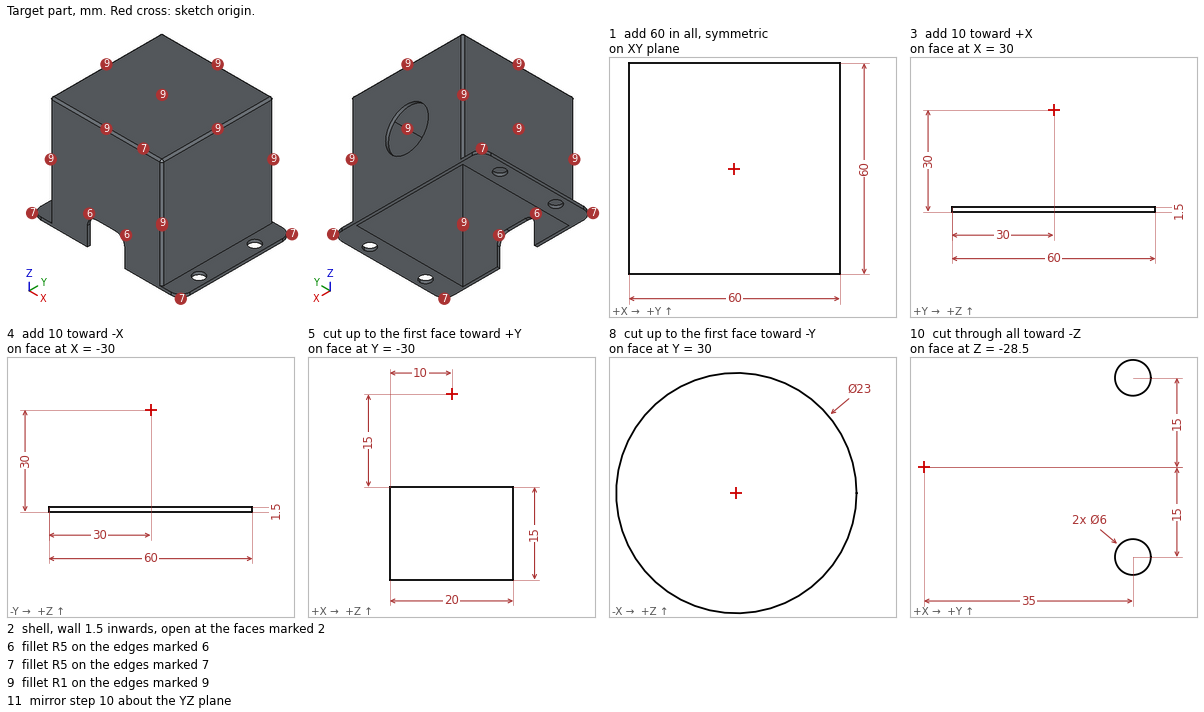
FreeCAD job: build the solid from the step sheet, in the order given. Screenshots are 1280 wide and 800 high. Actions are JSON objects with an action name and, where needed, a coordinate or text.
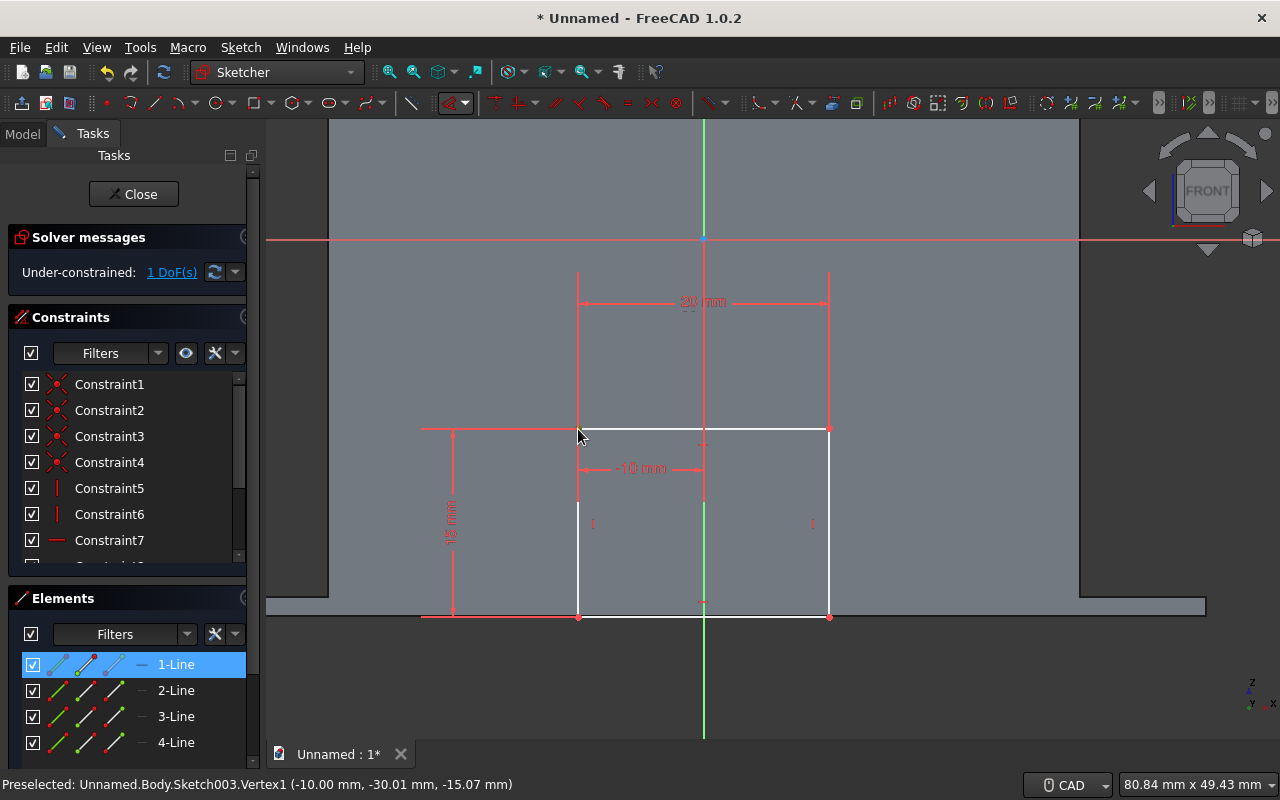
{"action": "left_click", "coordinate": [468, 104]}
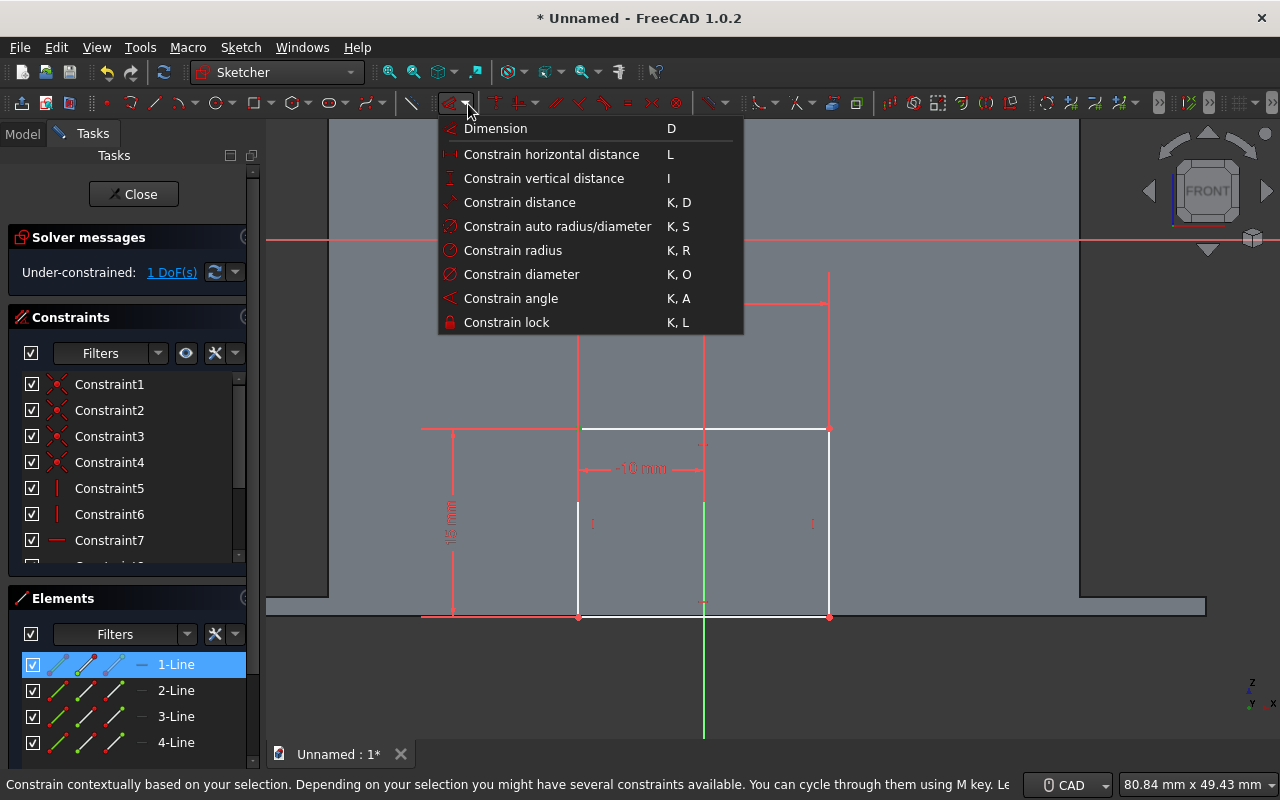
{"action": "left_click", "coordinate": [591, 178]}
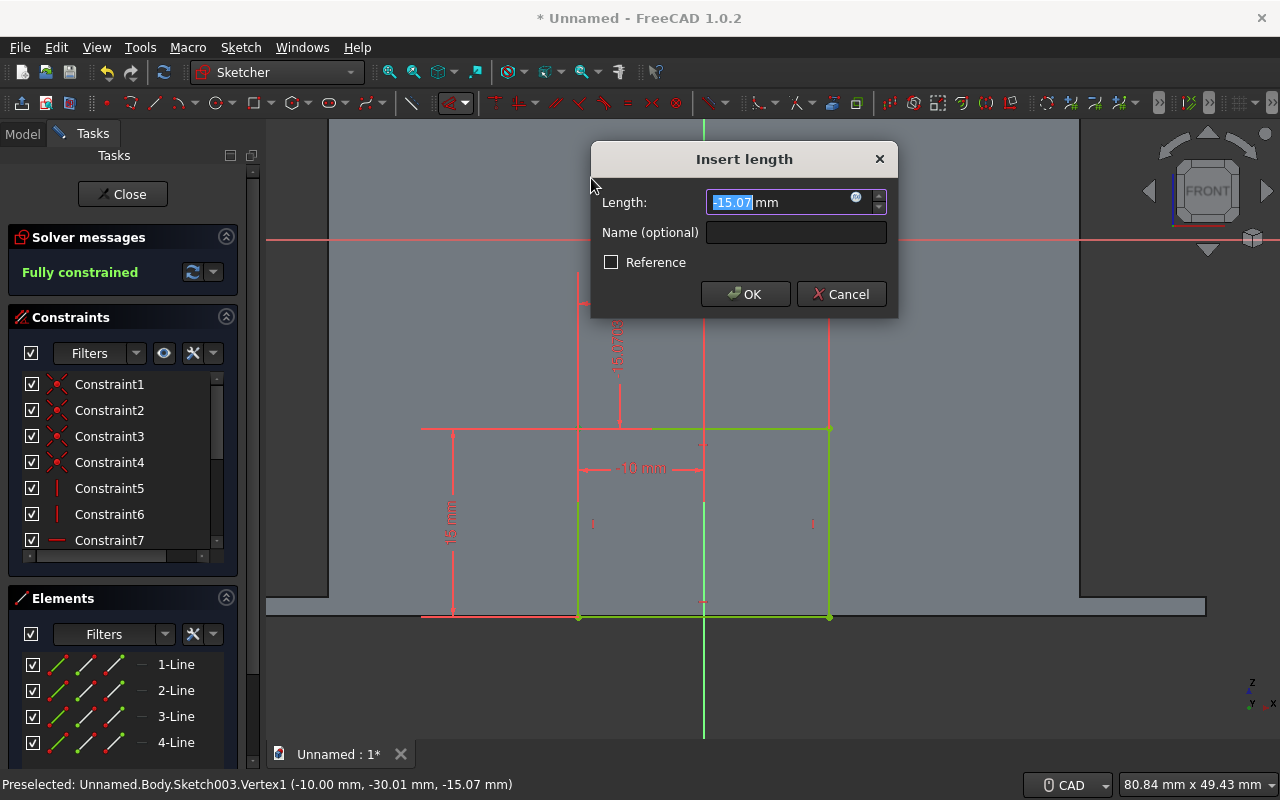
{"action": "type", "text": "-15"}
{"action": "key", "text": "Return"}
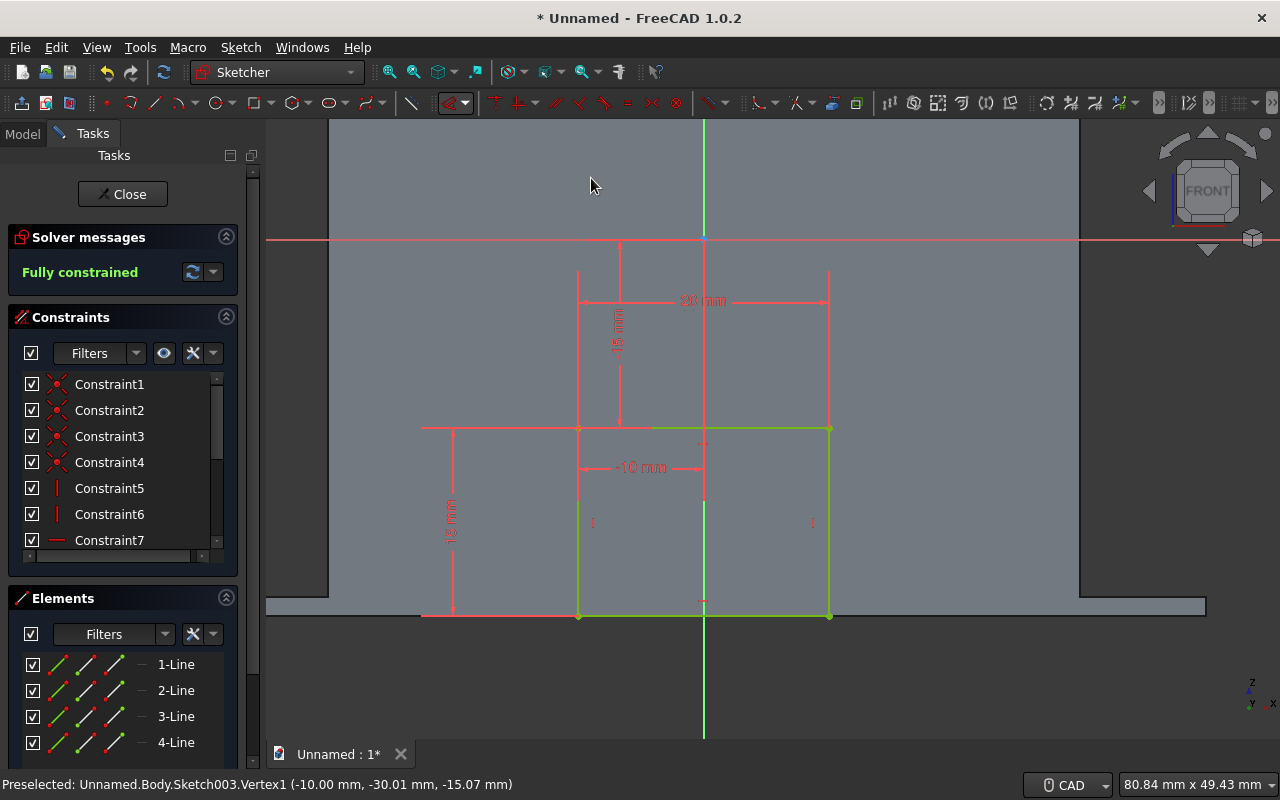
{"action": "left_click", "coordinate": [123, 194]}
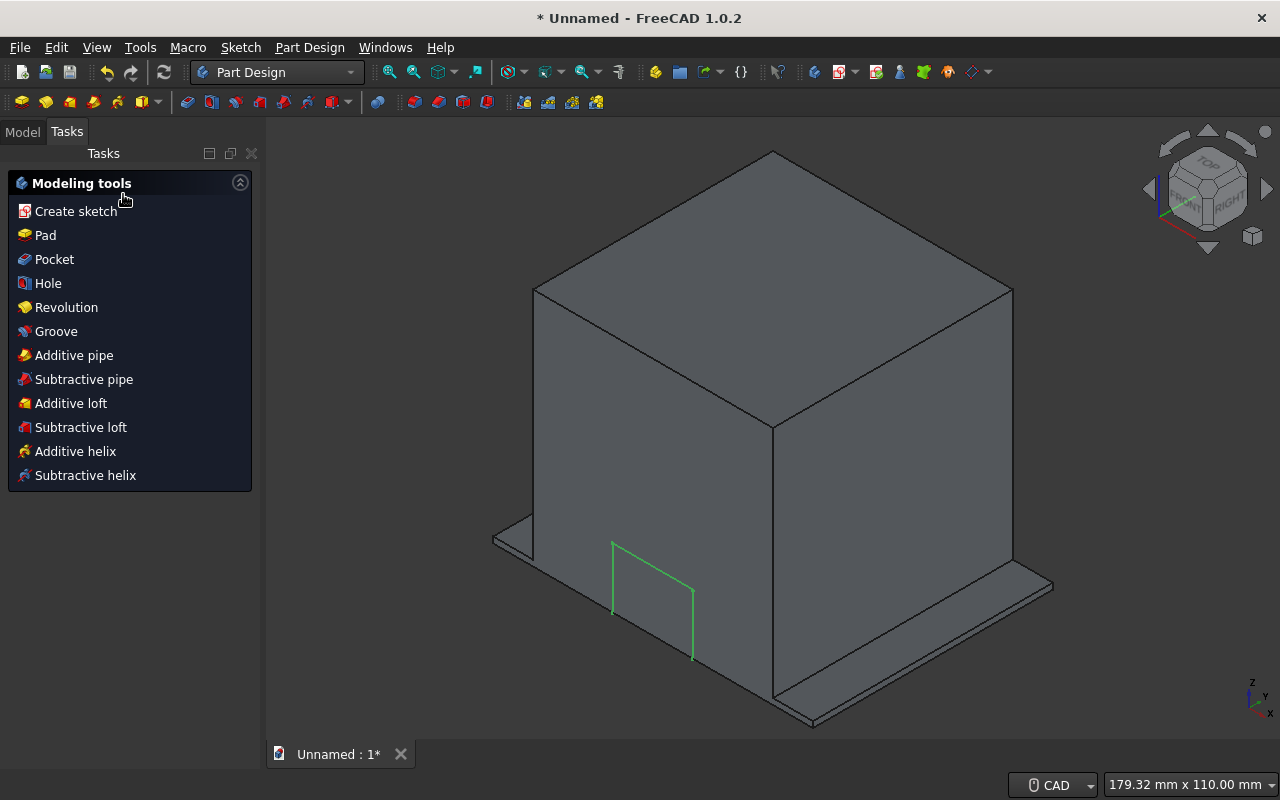
{"action": "left_click", "coordinate": [188, 102]}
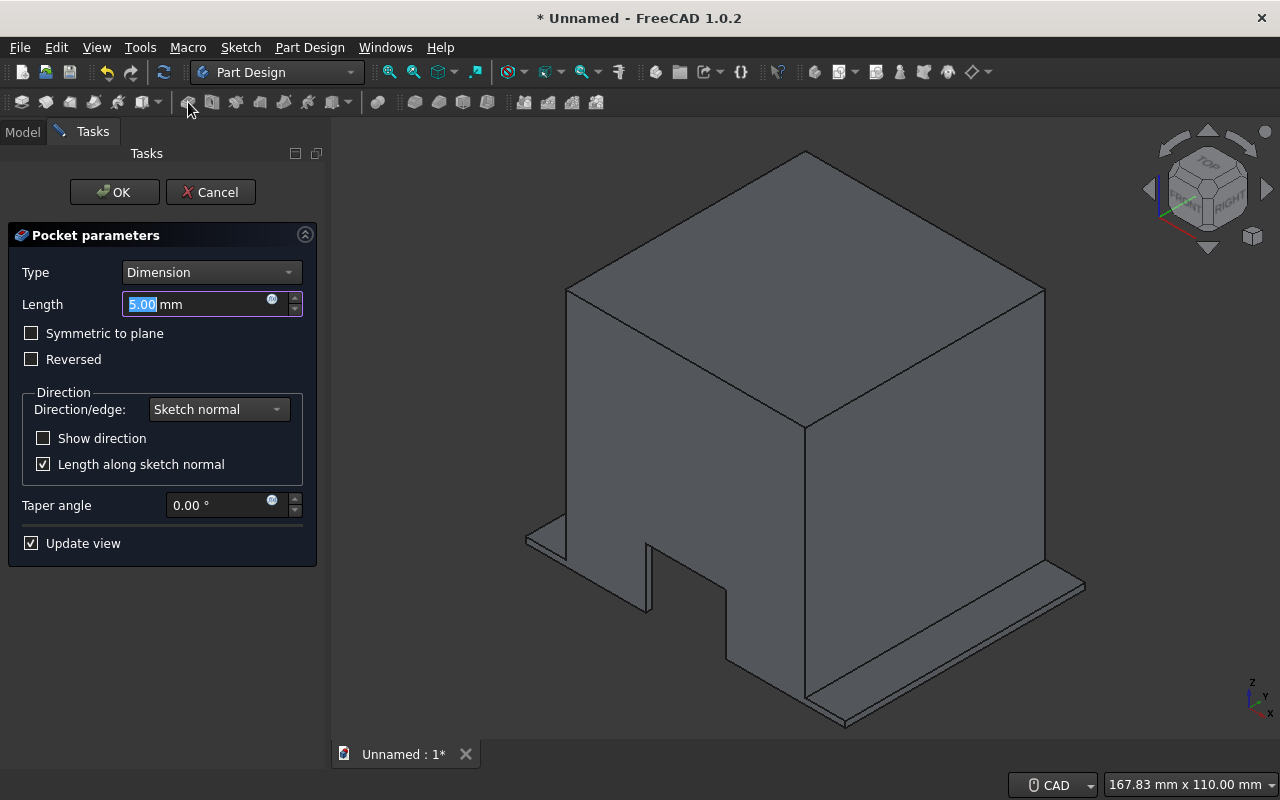
{"action": "left_click", "coordinate": [212, 272]}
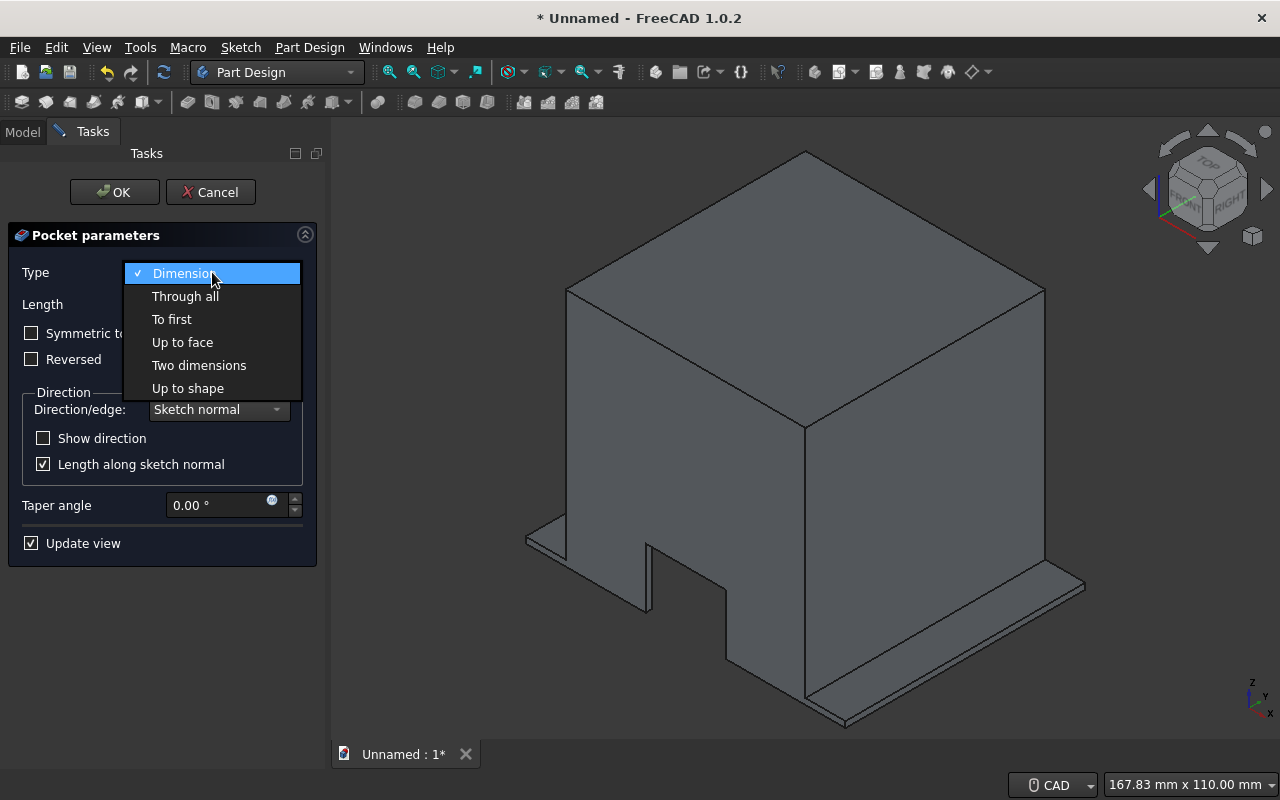
{"action": "left_click", "coordinate": [212, 320]}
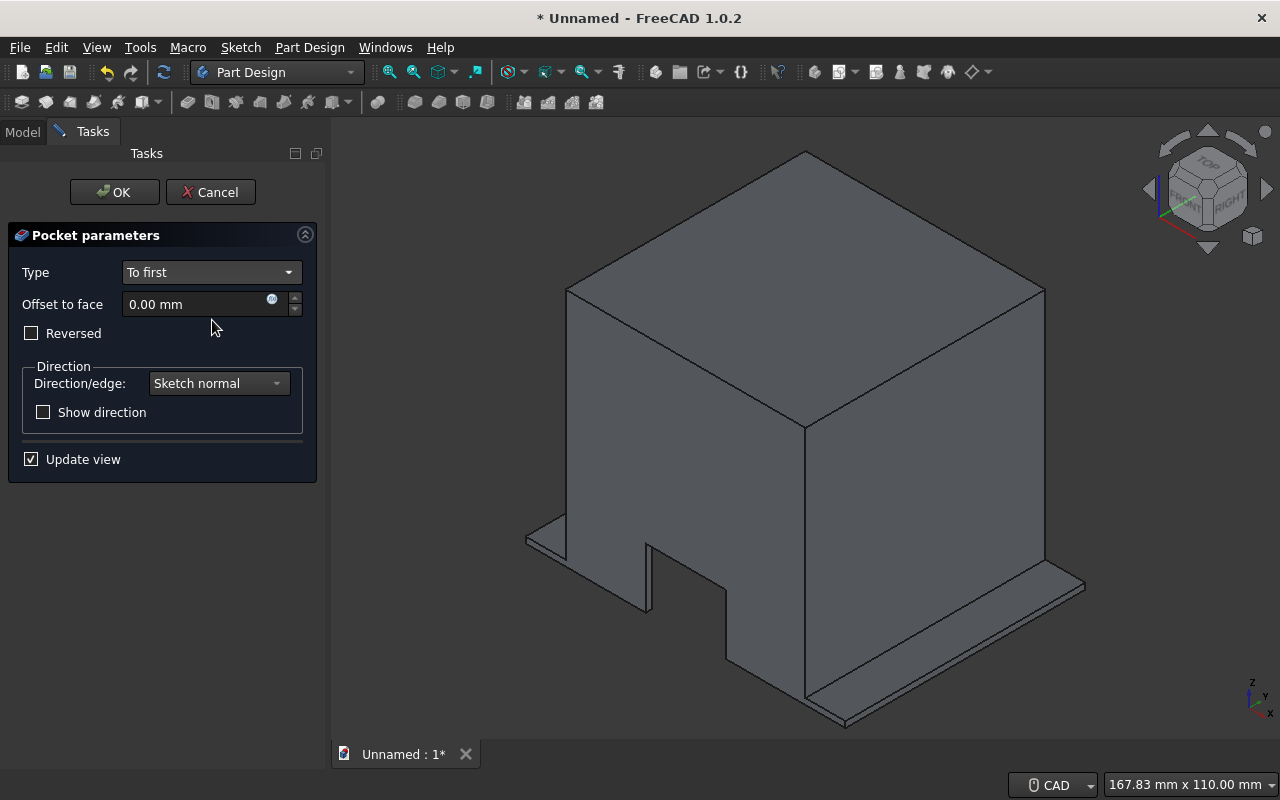
{"action": "left_click", "coordinate": [115, 192]}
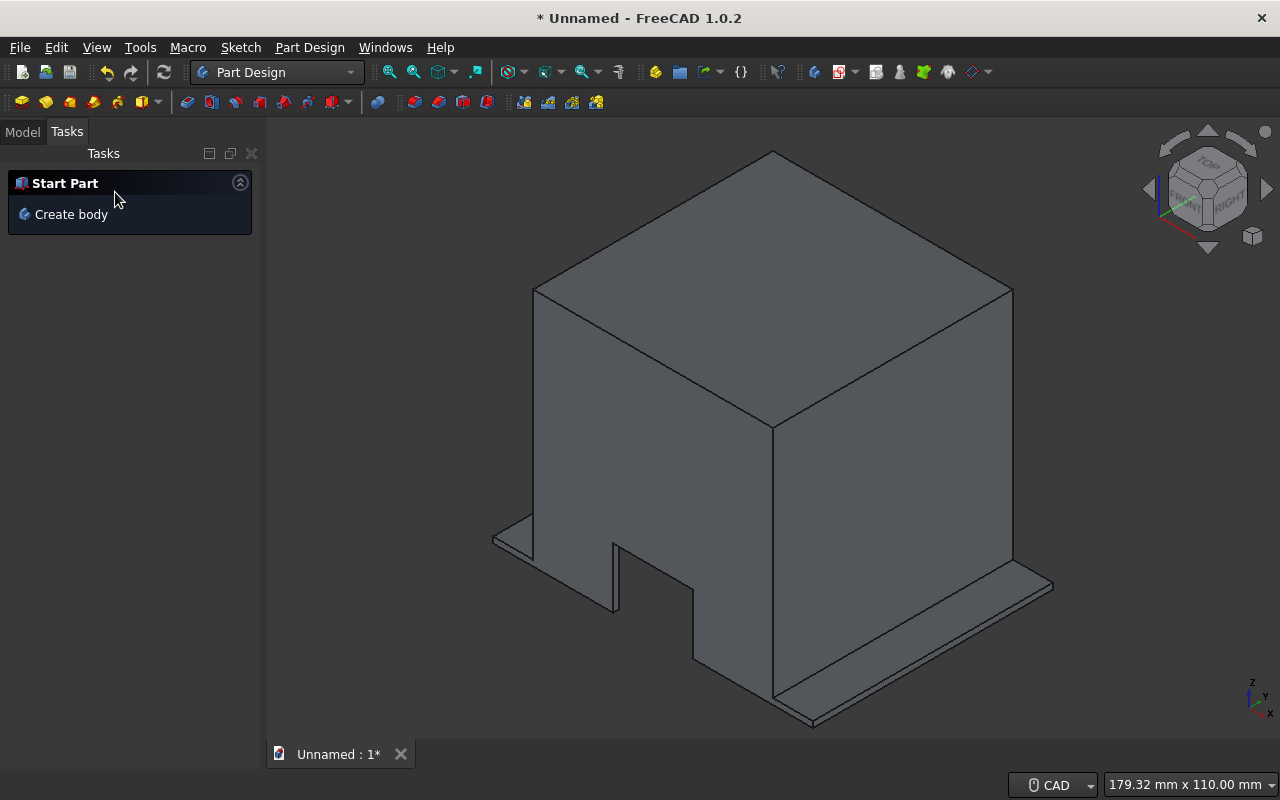
{"action": "scroll", "coordinate": [696, 587], "scroll_direction": "up", "scroll_amount": 8}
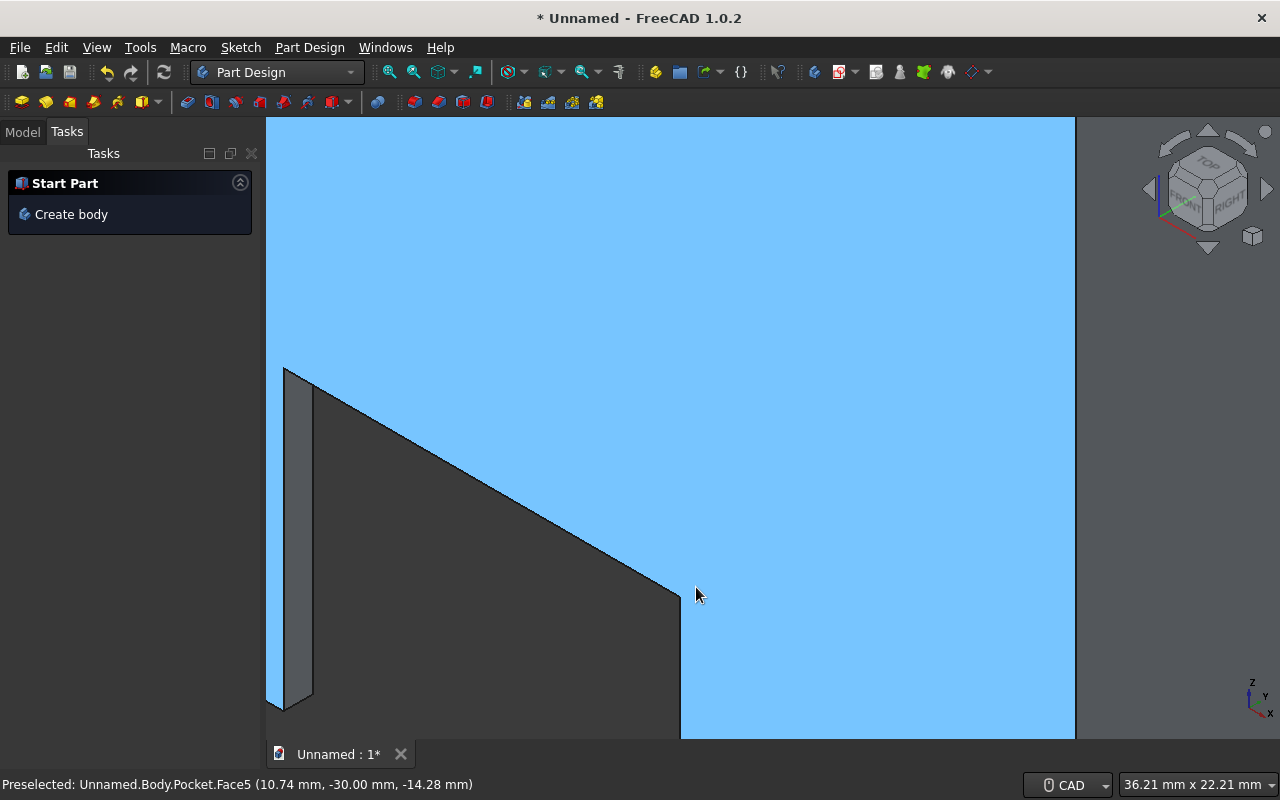
{"action": "left_click", "coordinate": [390, 72]}